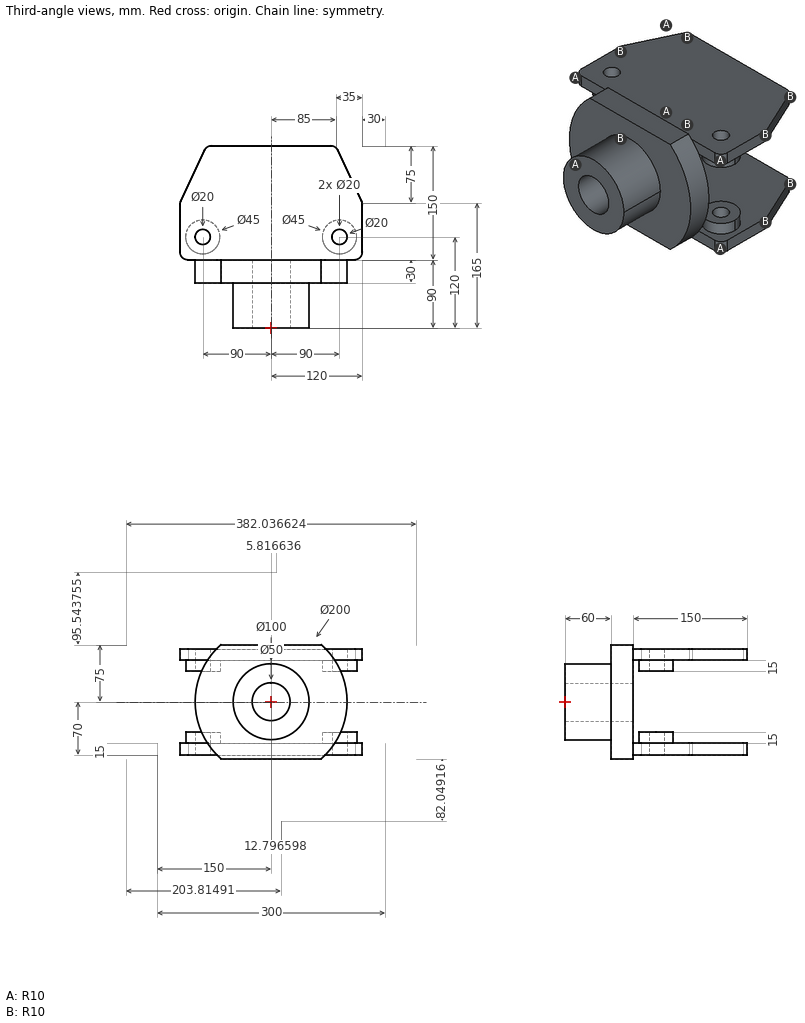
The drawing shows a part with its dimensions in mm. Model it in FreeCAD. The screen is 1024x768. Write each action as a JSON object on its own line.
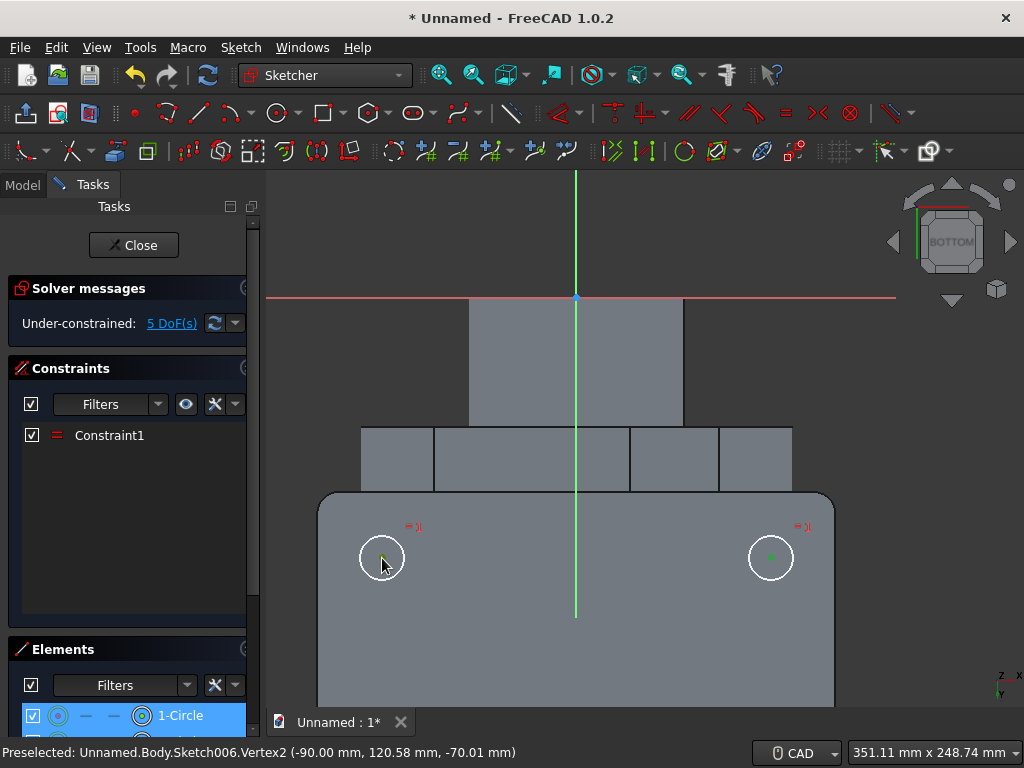
{"action": "left_click", "coordinate": [576, 610]}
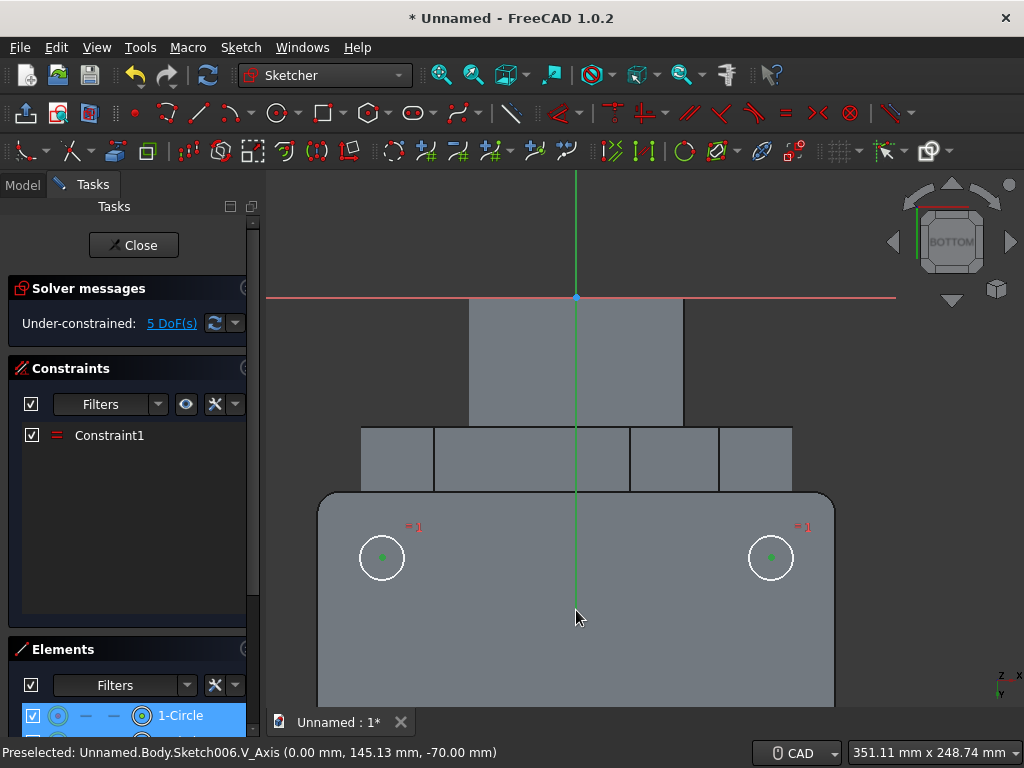
{"action": "left_click", "coordinate": [818, 114]}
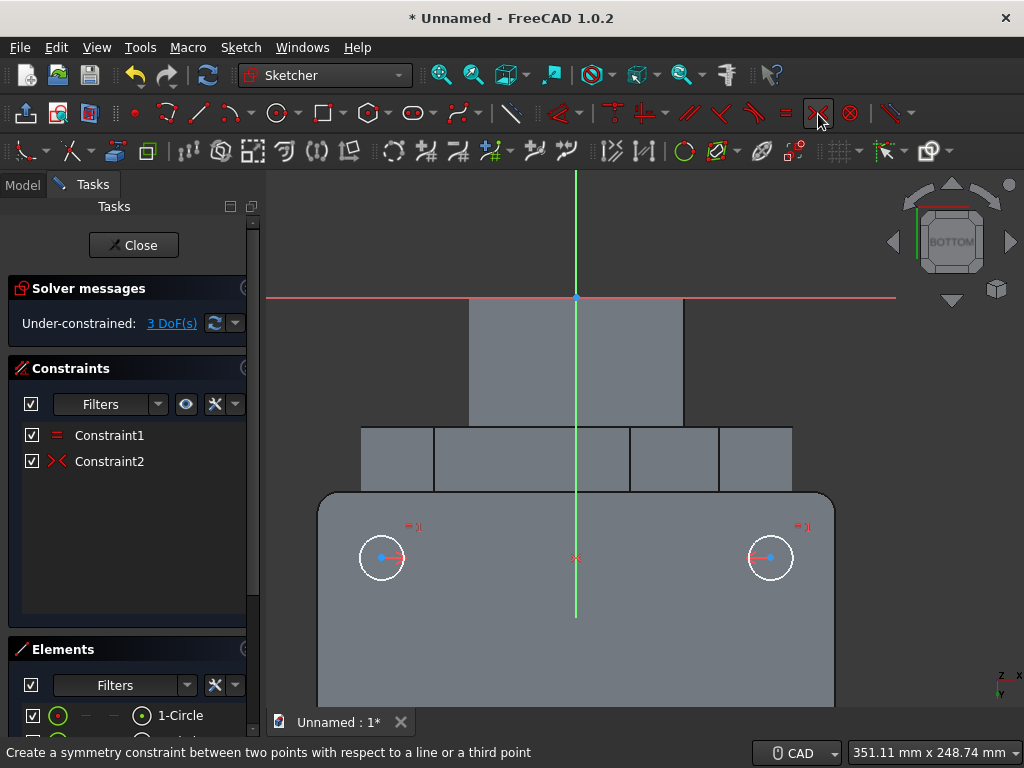
{"action": "left_click", "coordinate": [558, 114]}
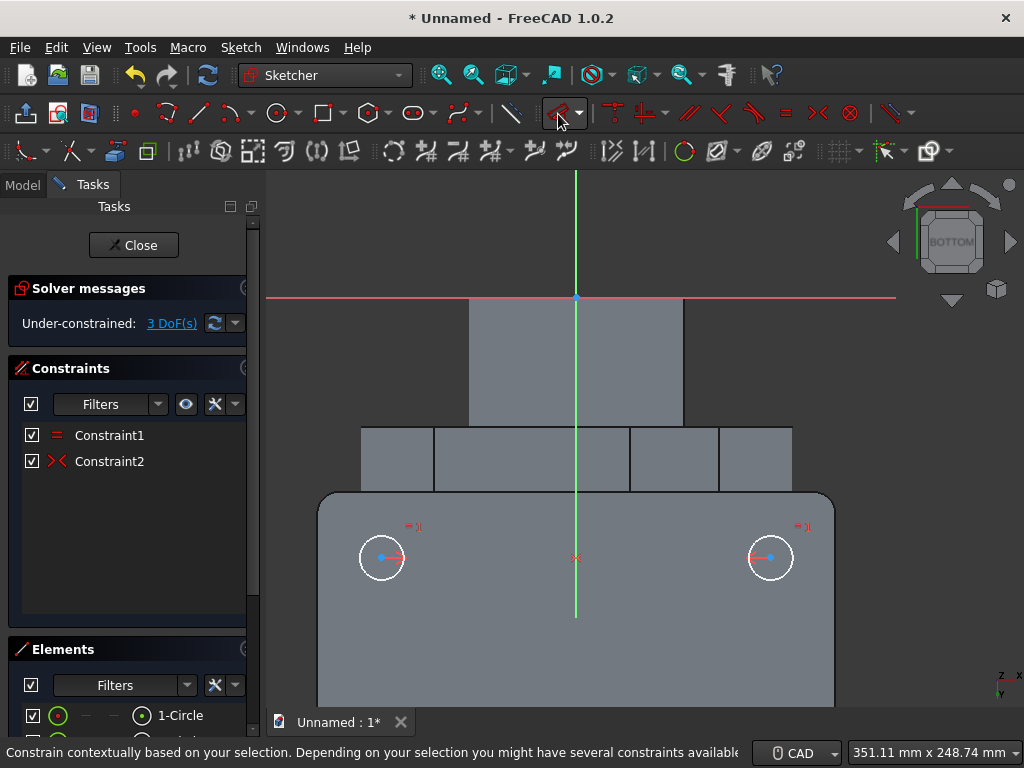
{"action": "left_click", "coordinate": [786, 542]}
{"action": "left_click", "coordinate": [808, 519]}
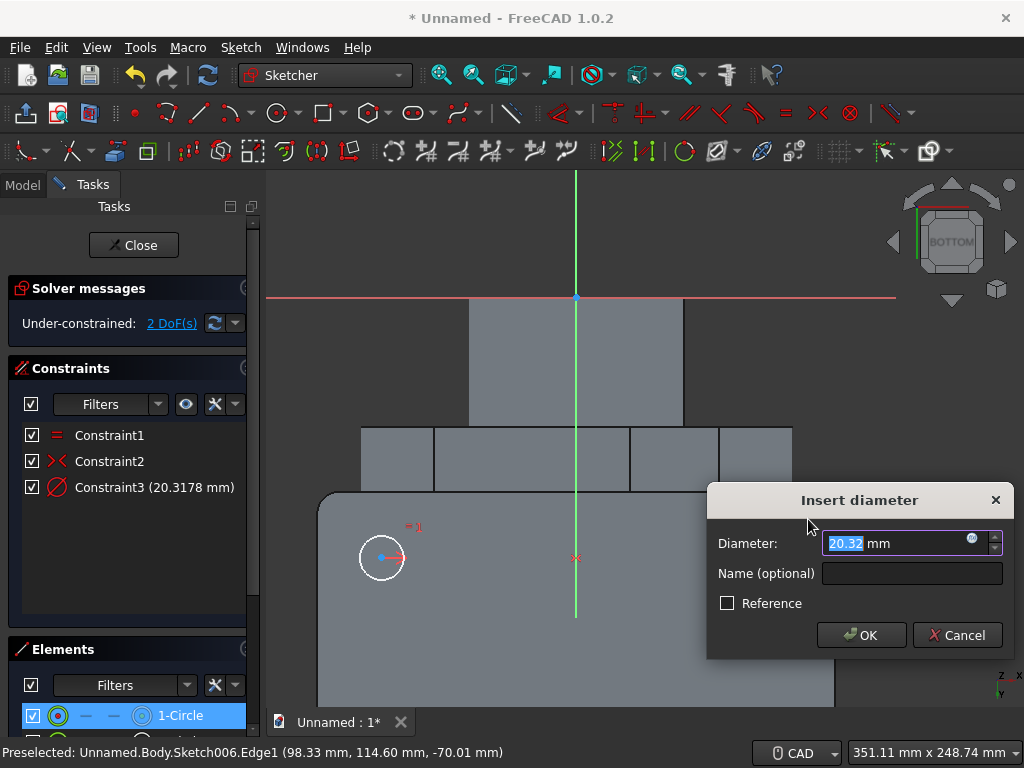
{"action": "type", "text": "20"}
{"action": "key", "text": "Return"}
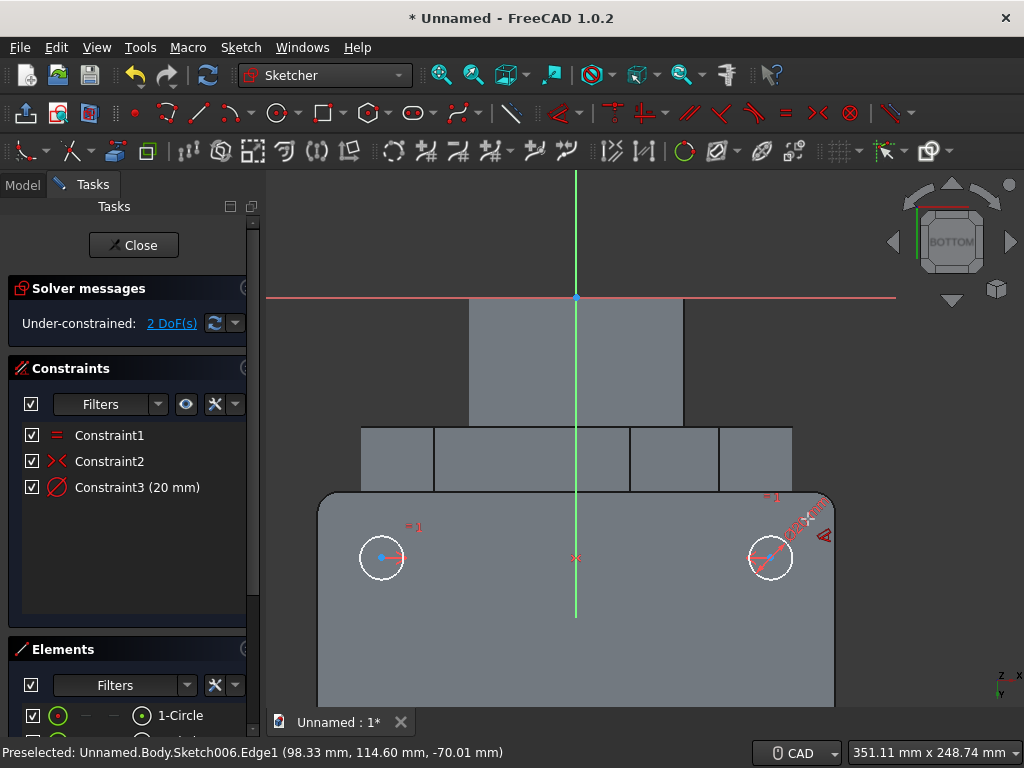
{"action": "left_click", "coordinate": [771, 558]}
{"action": "left_click", "coordinate": [674, 264]}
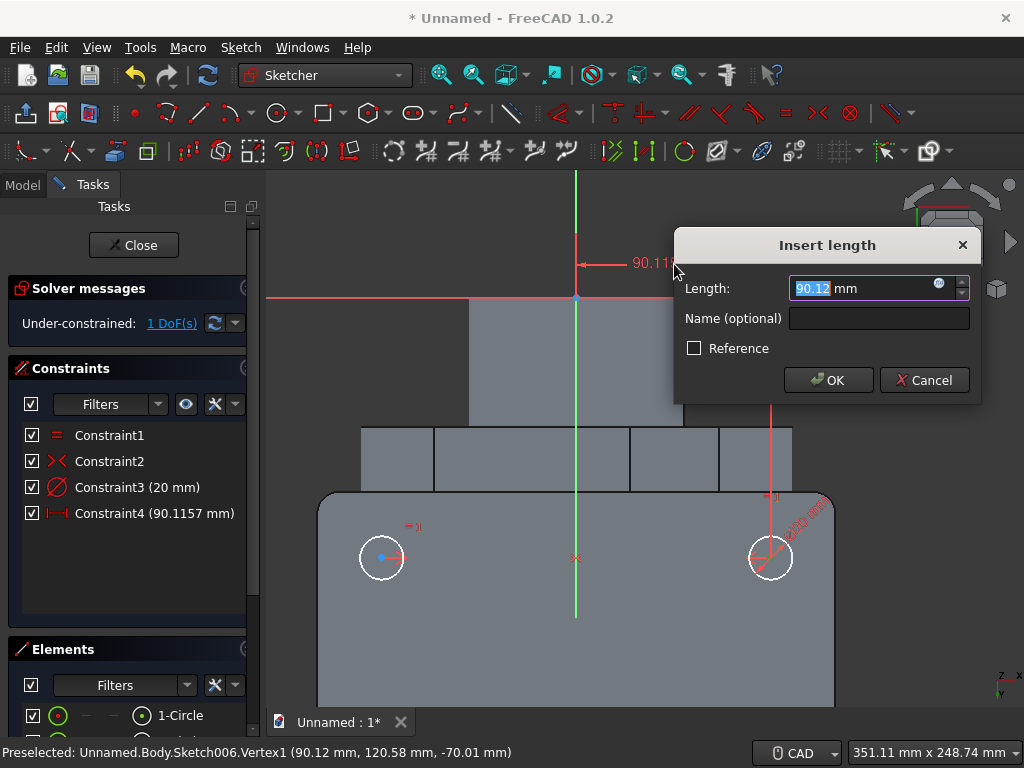
{"action": "type", "text": "90"}
{"action": "key", "text": "Return"}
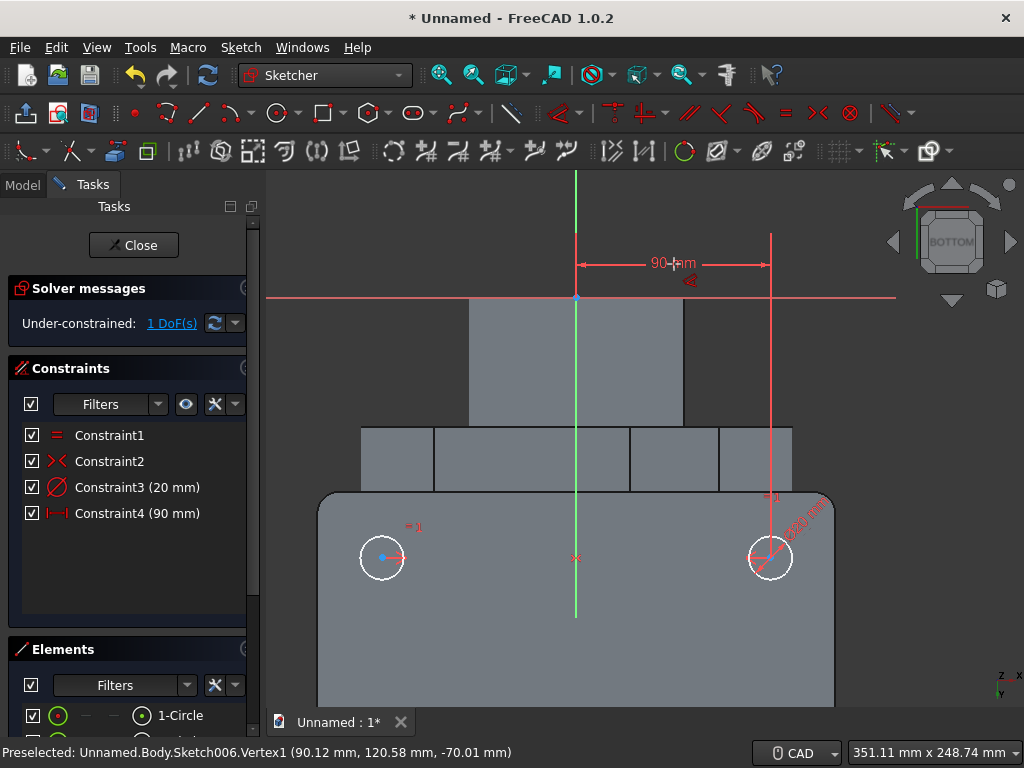
{"action": "left_click", "coordinate": [771, 558]}
{"action": "left_click", "coordinate": [805, 428]}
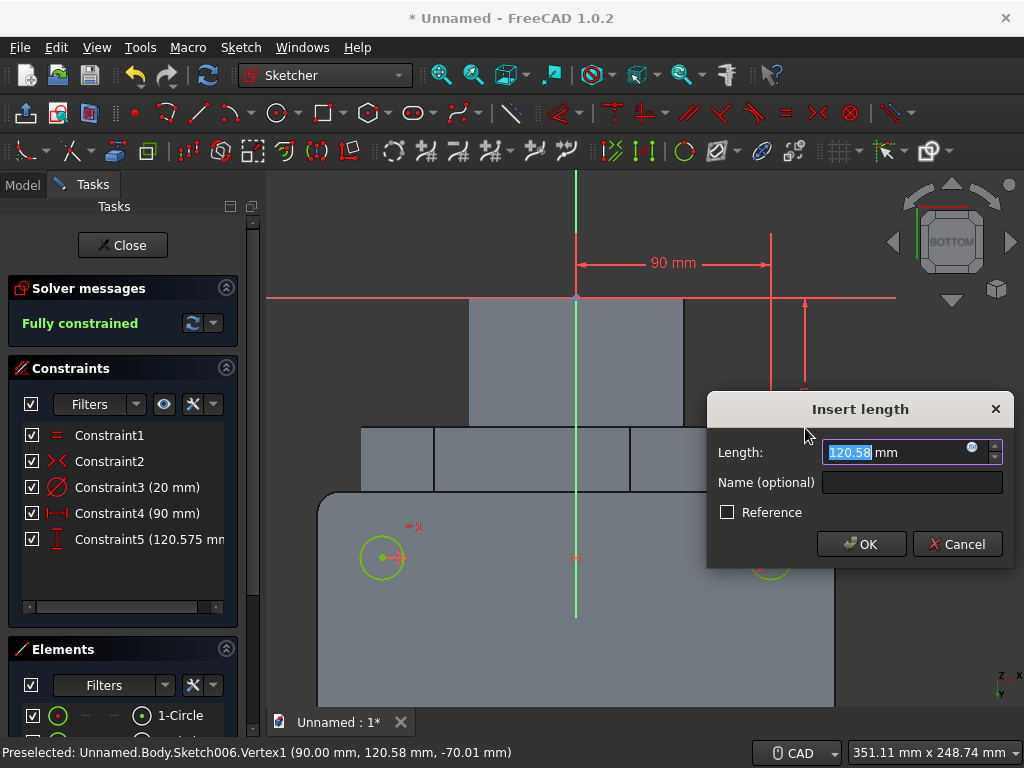
{"action": "type", "text": "120"}
{"action": "key", "text": "Return"}
{"action": "key", "text": "Escape"}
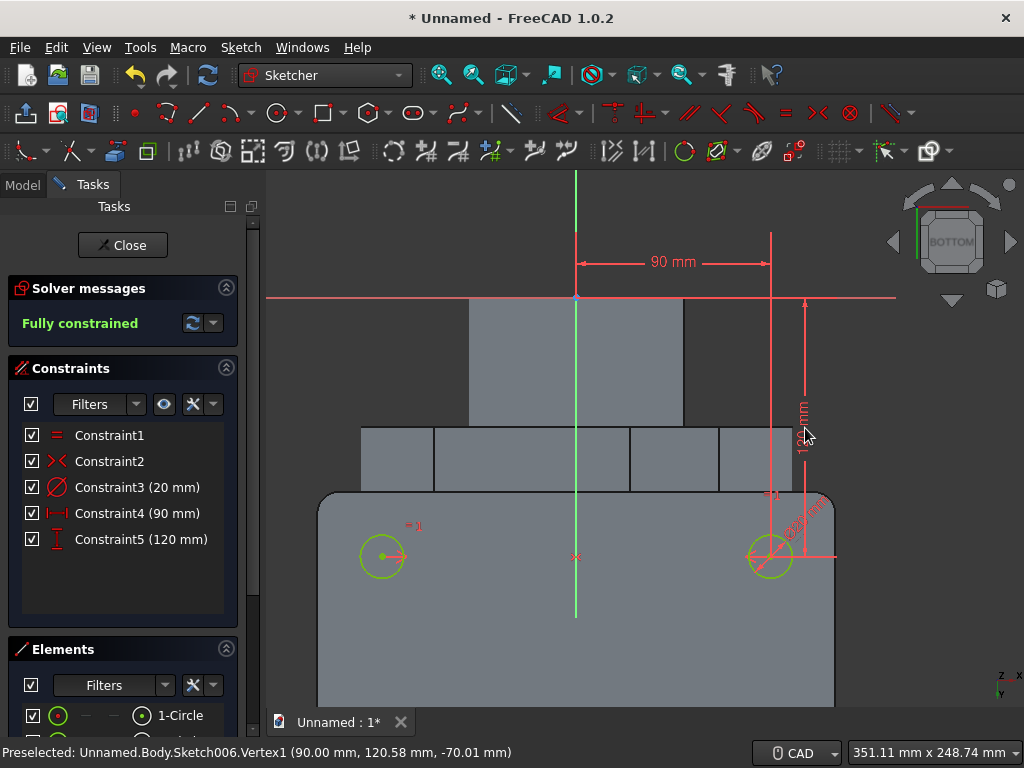
{"action": "left_click", "coordinate": [123, 245]}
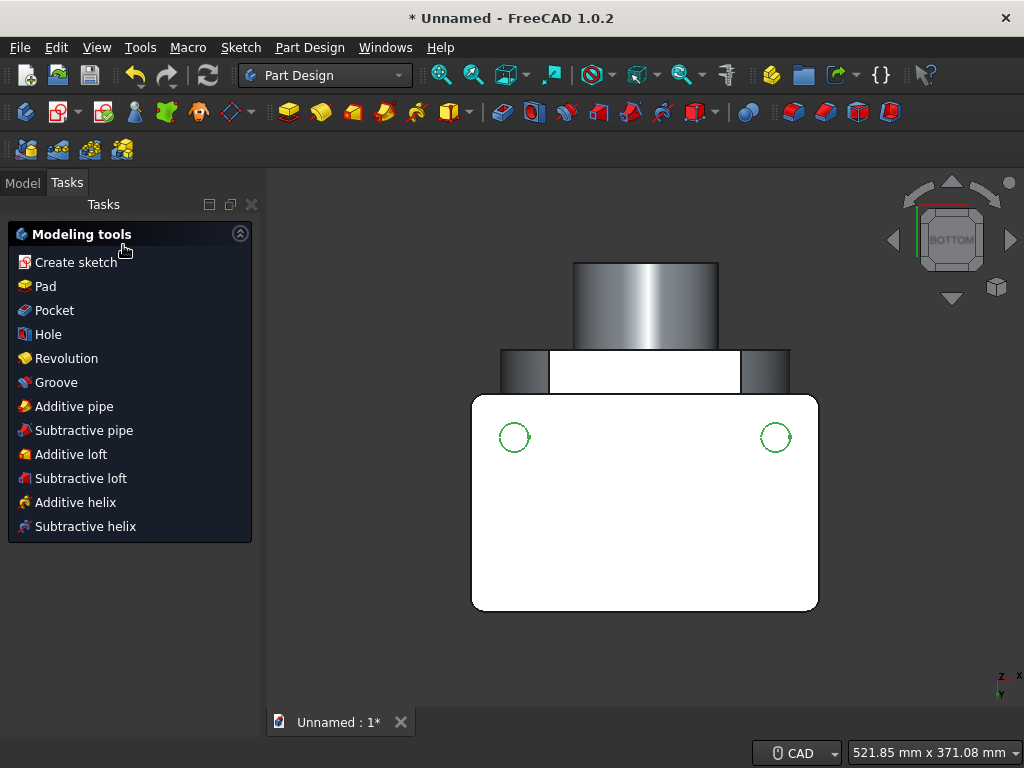
{"action": "left_click", "coordinate": [504, 112]}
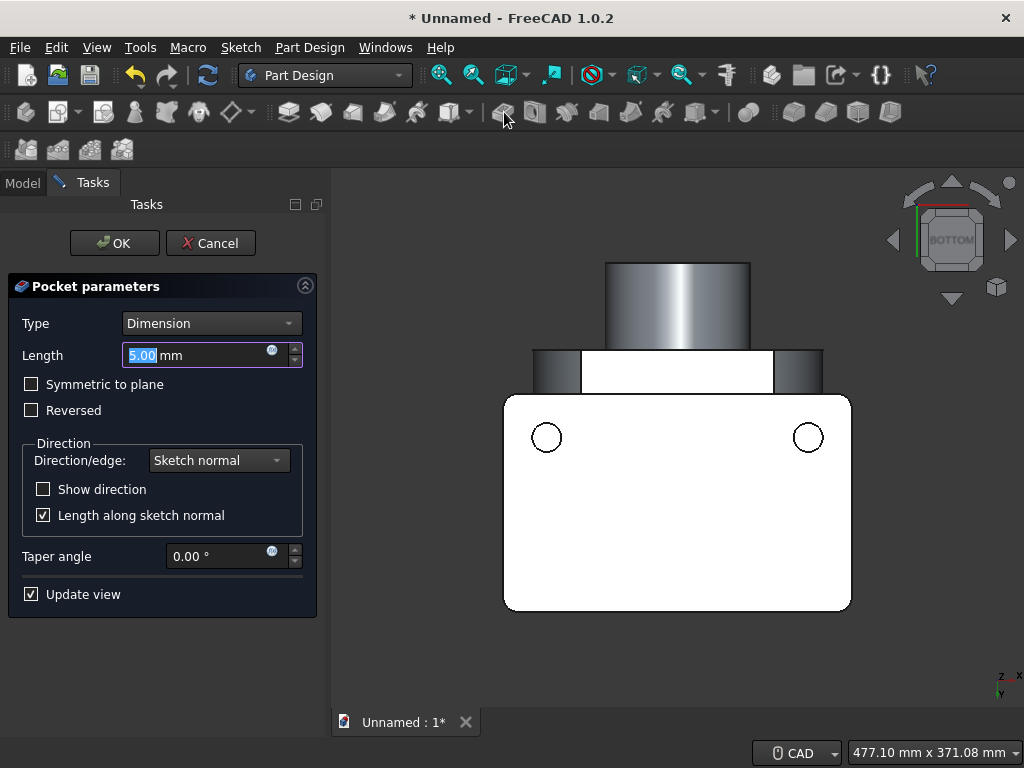
{"action": "left_click", "coordinate": [212, 324]}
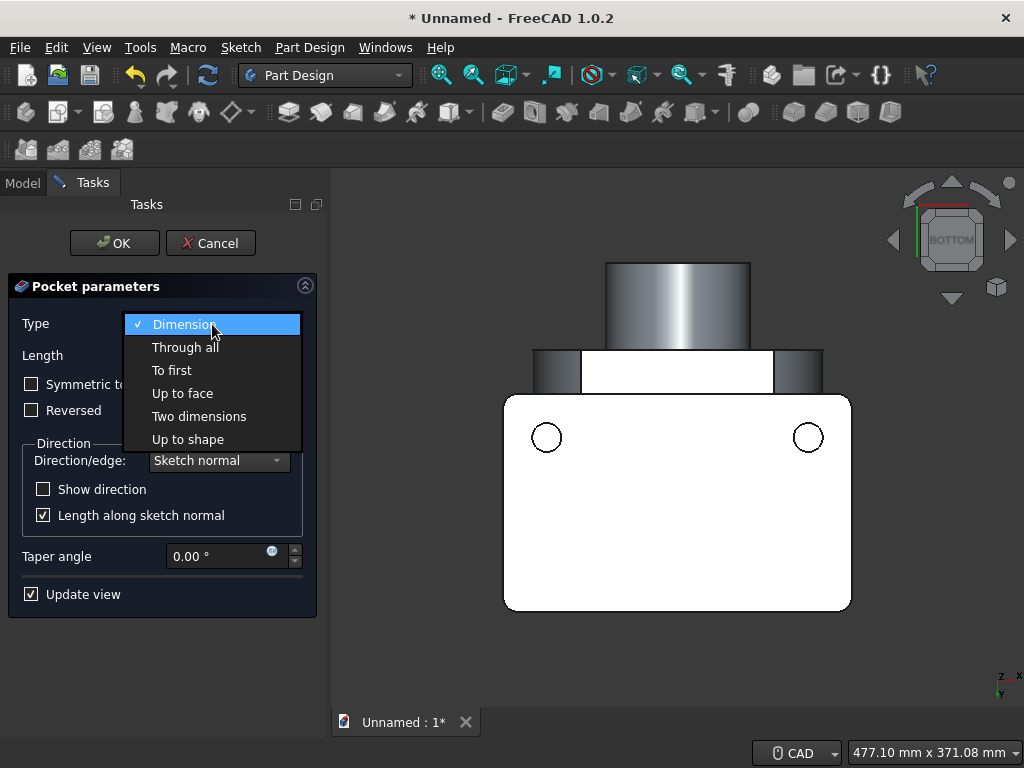
{"action": "left_click", "coordinate": [212, 348]}